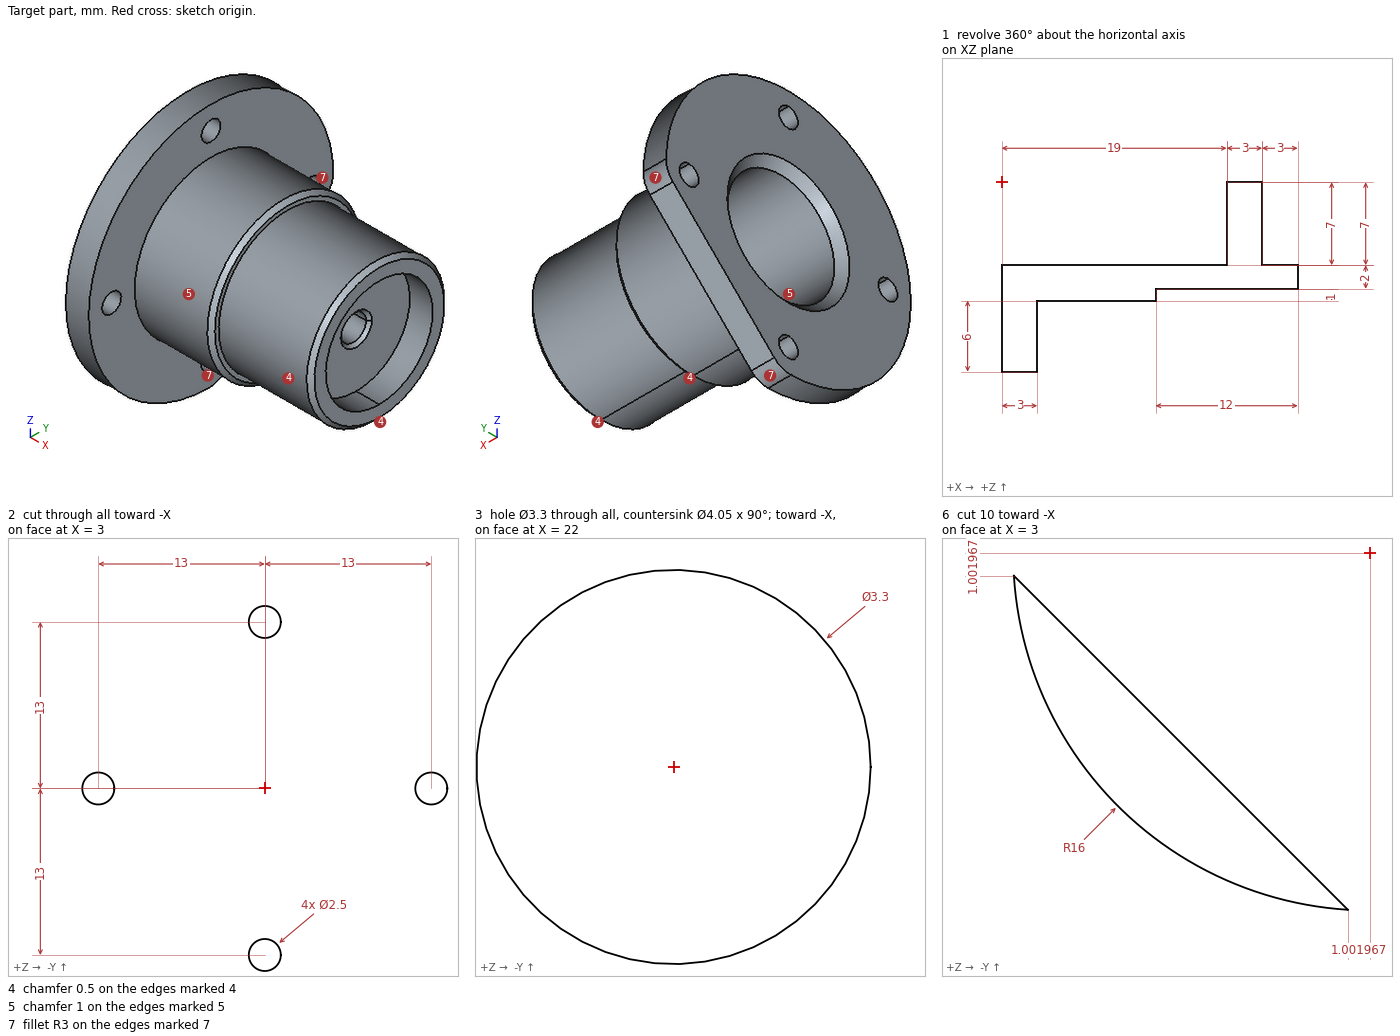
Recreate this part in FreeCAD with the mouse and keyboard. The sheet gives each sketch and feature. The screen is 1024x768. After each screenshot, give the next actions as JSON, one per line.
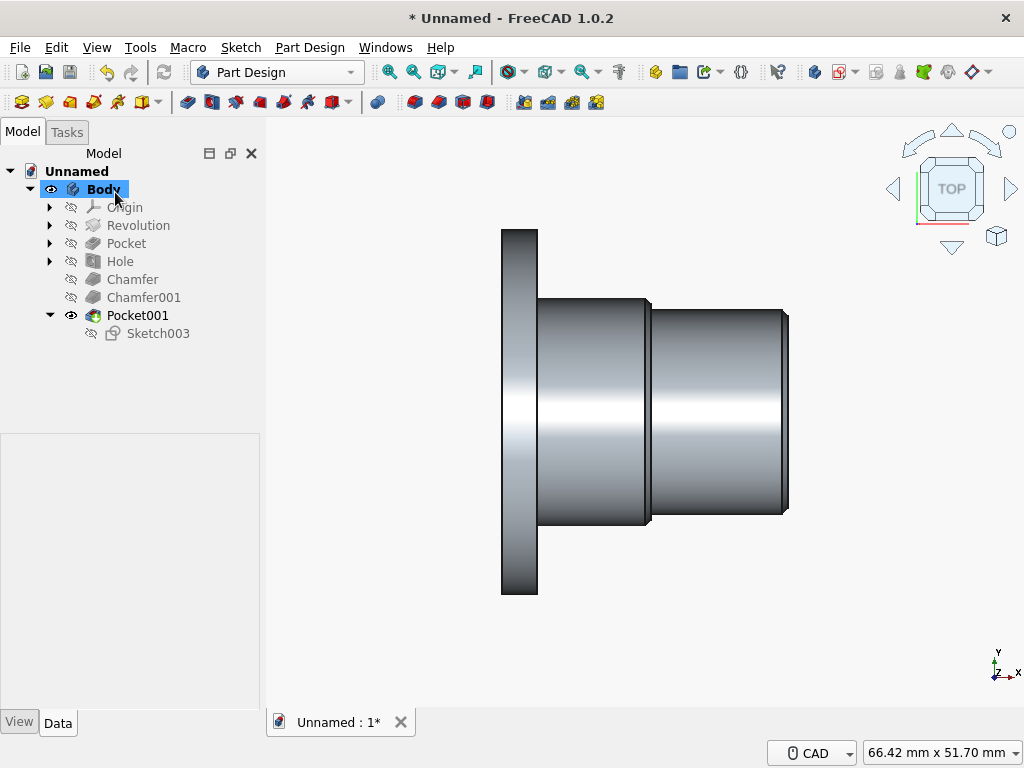
{"action": "key", "text": "0"}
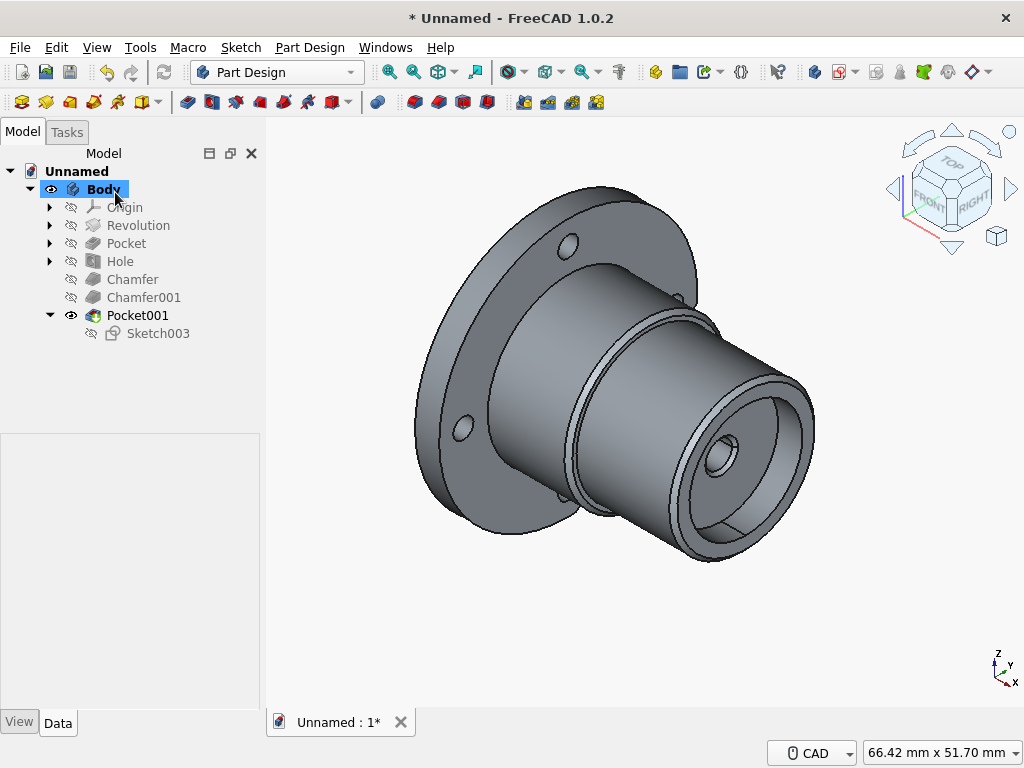
{"action": "key", "text": "1"}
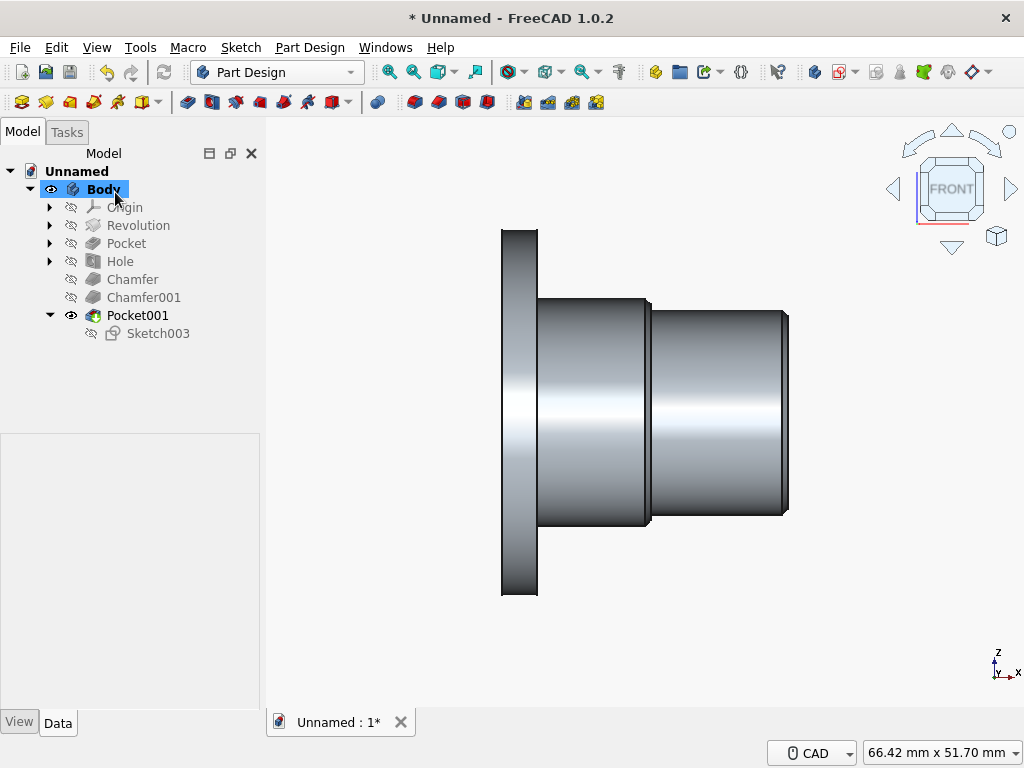
{"action": "key", "text": "3"}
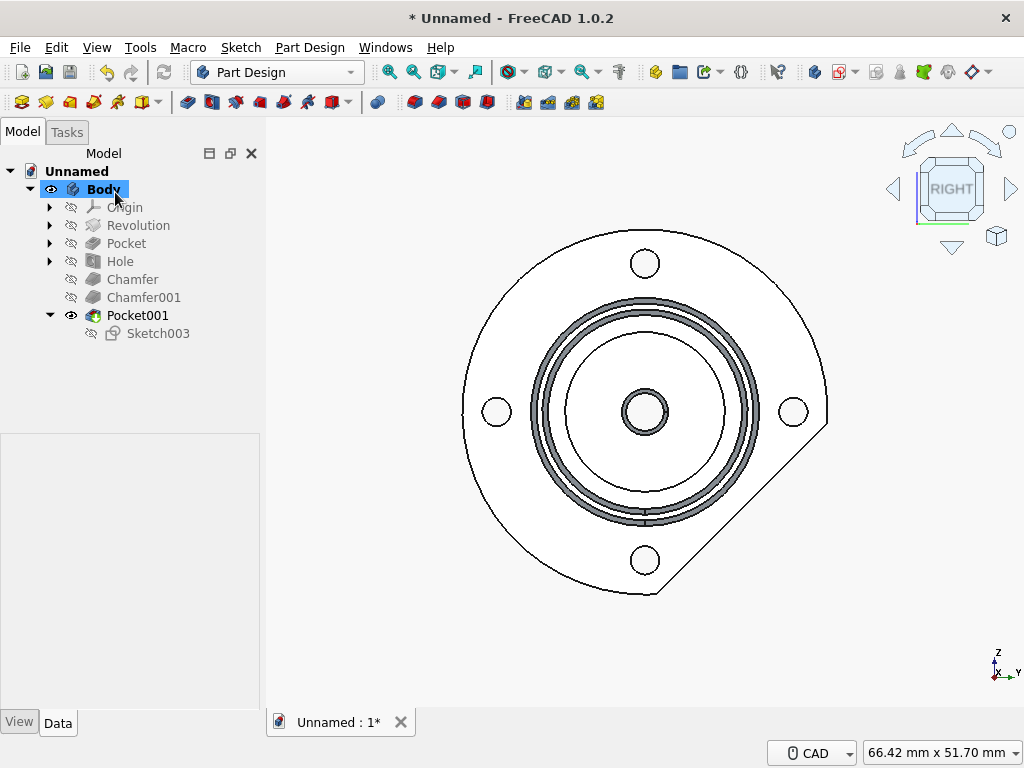
{"action": "key", "text": "5"}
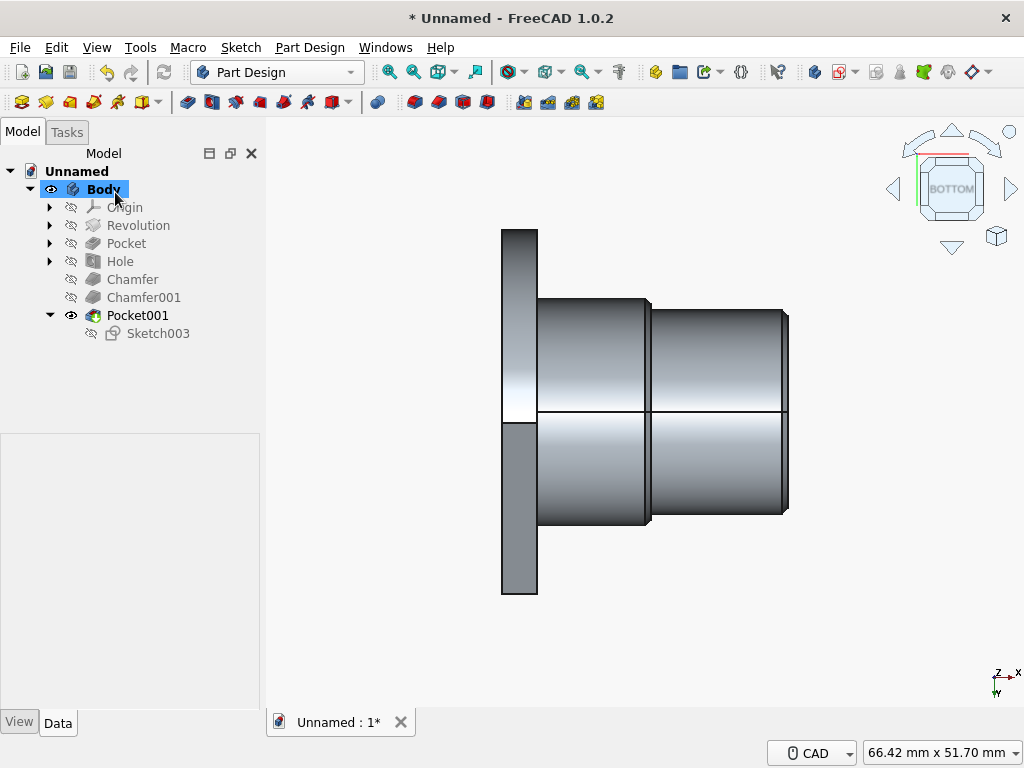
{"action": "key", "text": "4"}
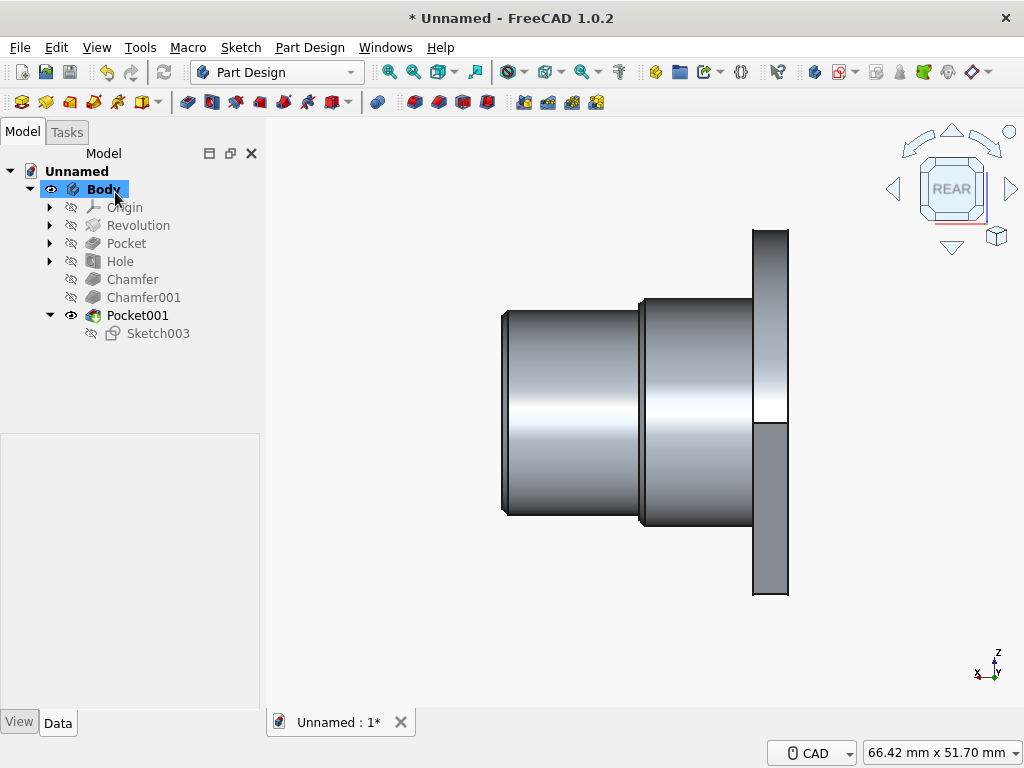
{"action": "key", "text": "6"}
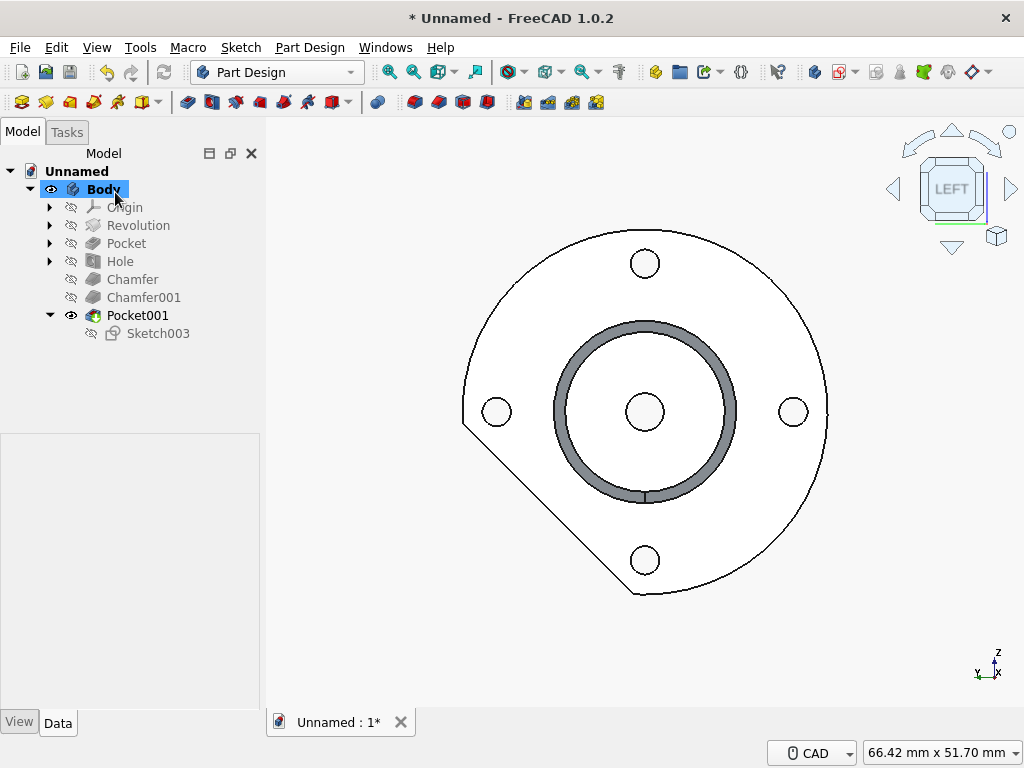
{"action": "key", "text": "v 3"}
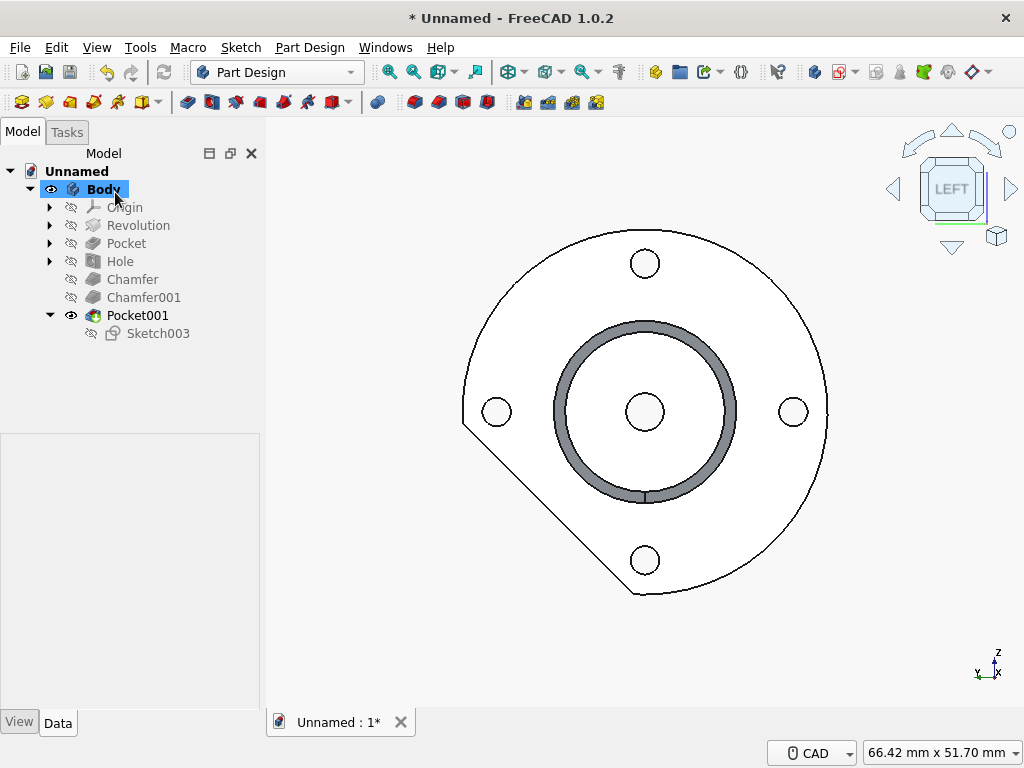
{"action": "key", "text": "0"}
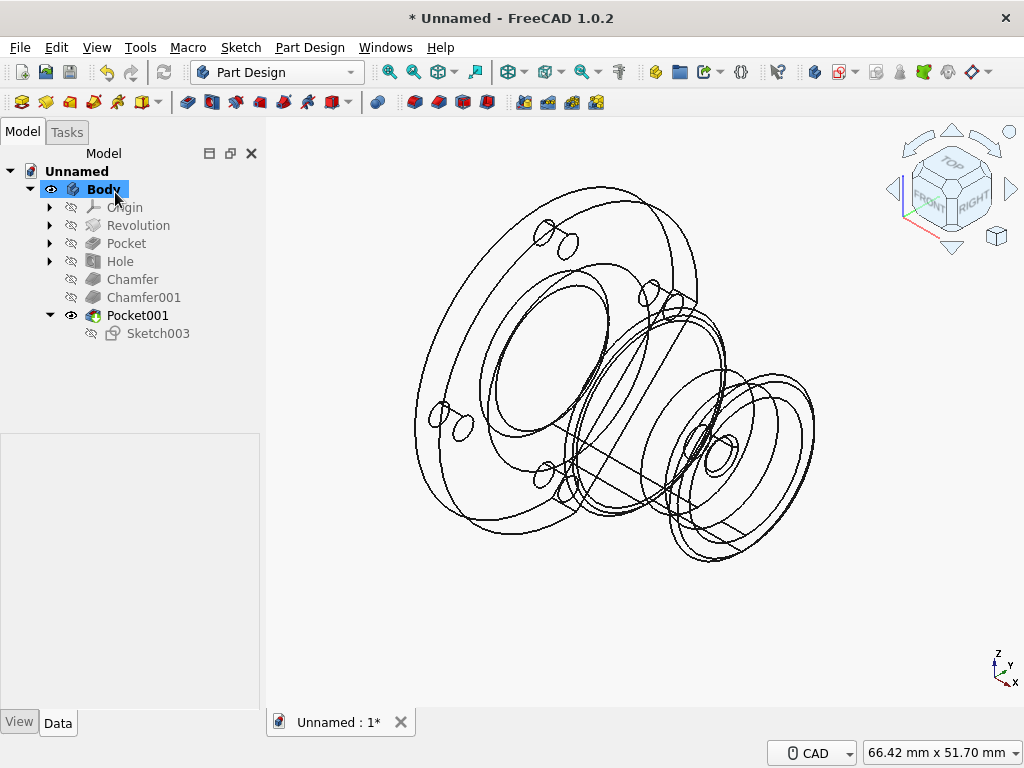
{"action": "left_click", "coordinate": [690, 297]}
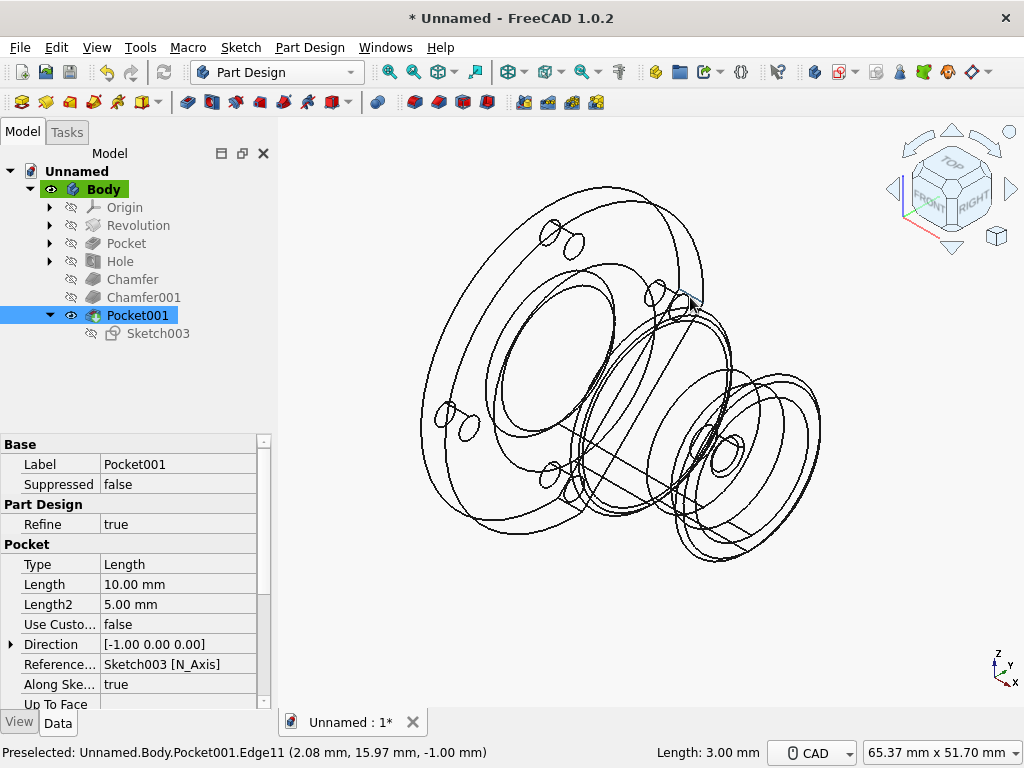
{"action": "left_click", "coordinate": [575, 507], "text": "ctrl"}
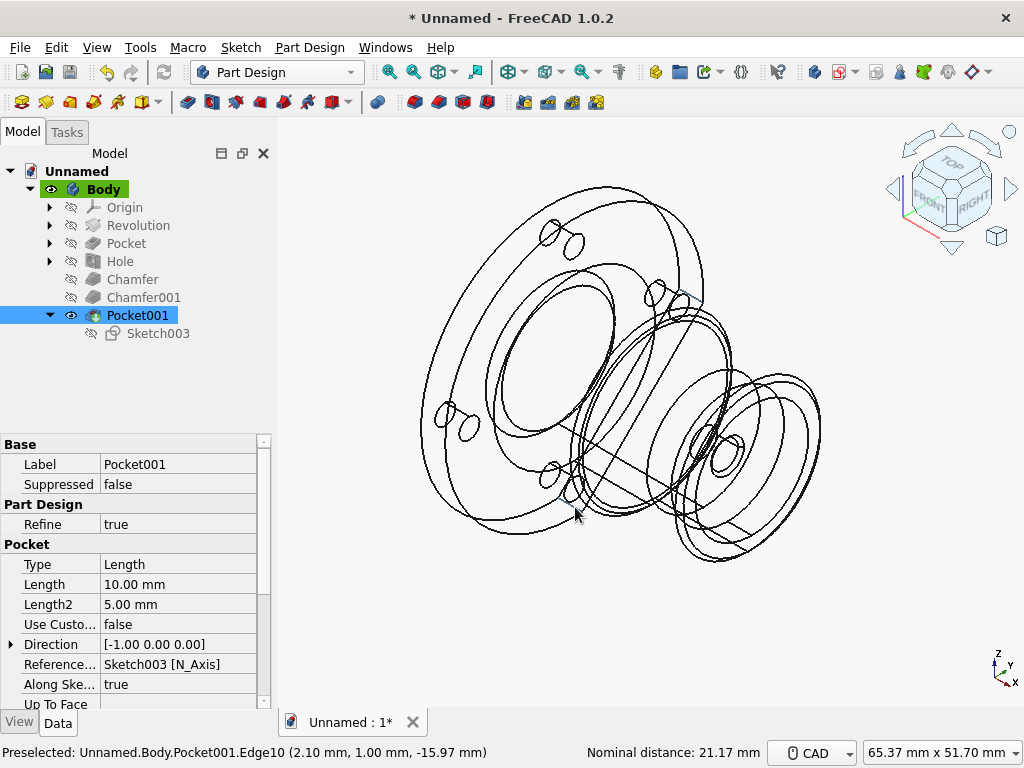
{"action": "key", "text": "v 1"}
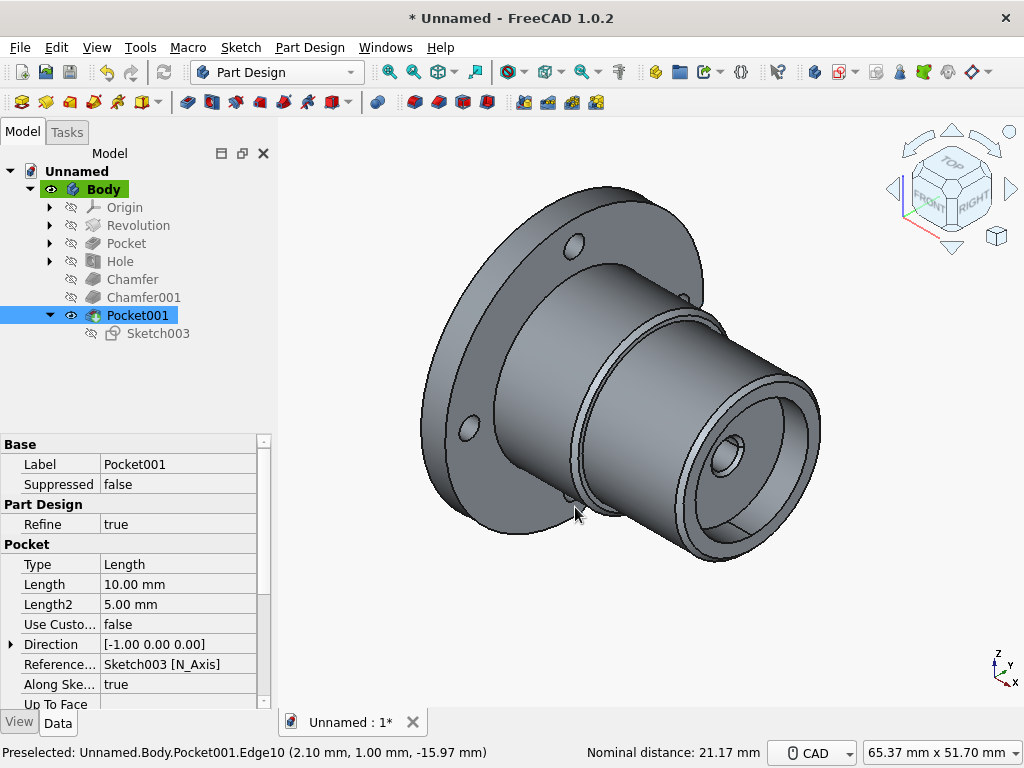
{"action": "left_click", "coordinate": [416, 102]}